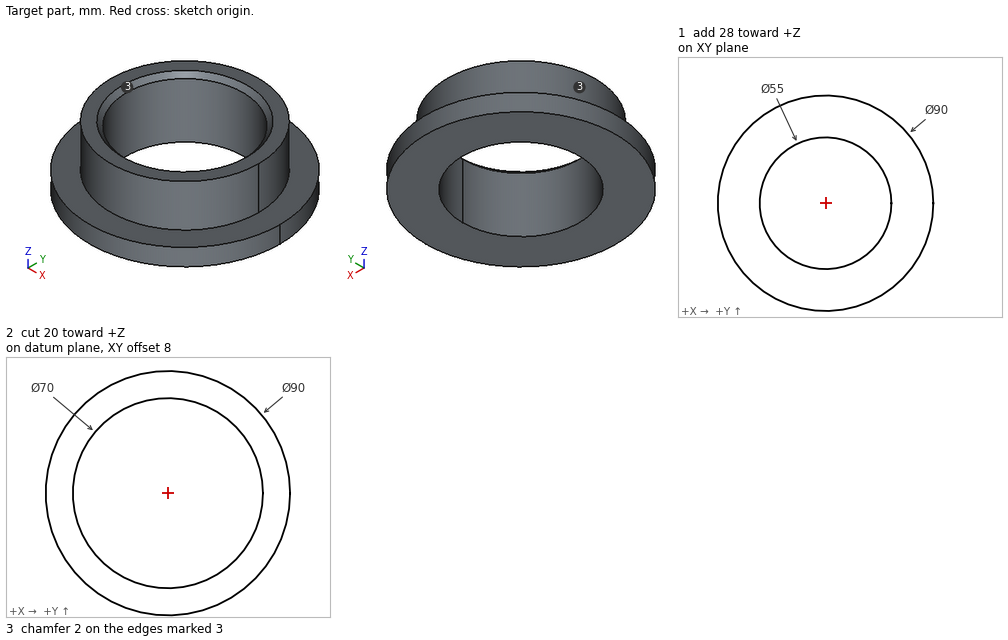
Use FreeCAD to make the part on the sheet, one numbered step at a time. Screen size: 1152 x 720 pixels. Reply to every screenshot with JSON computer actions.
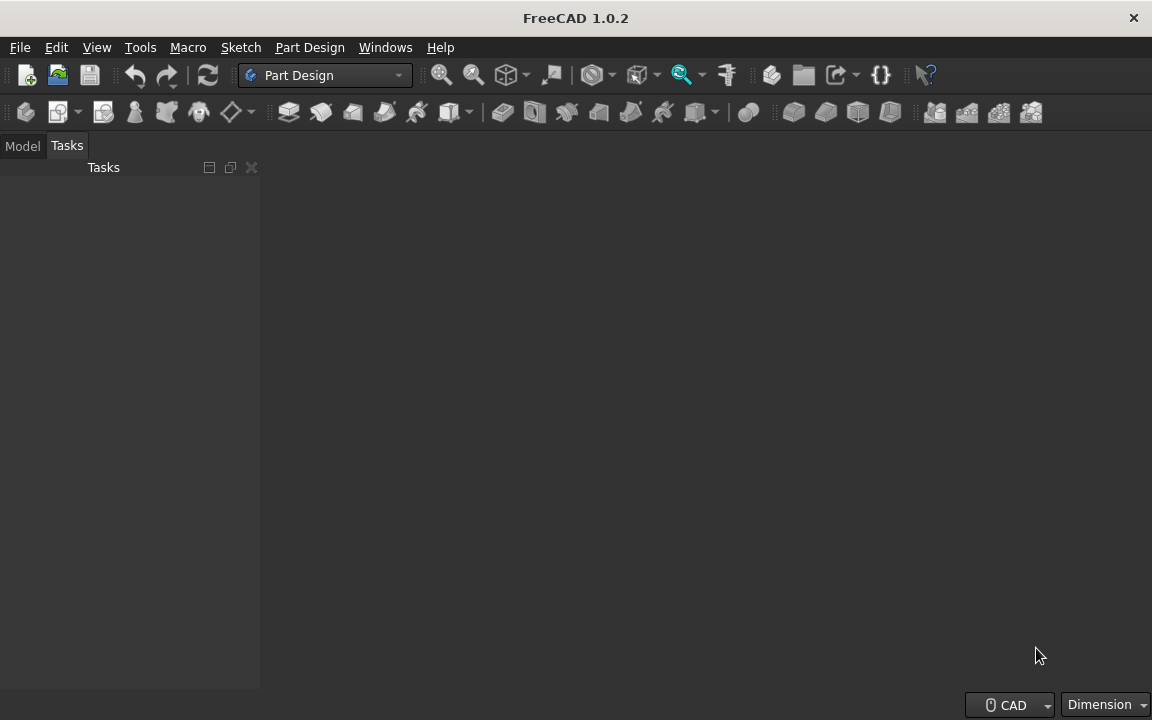
{"action": "left_click", "coordinate": [26, 76]}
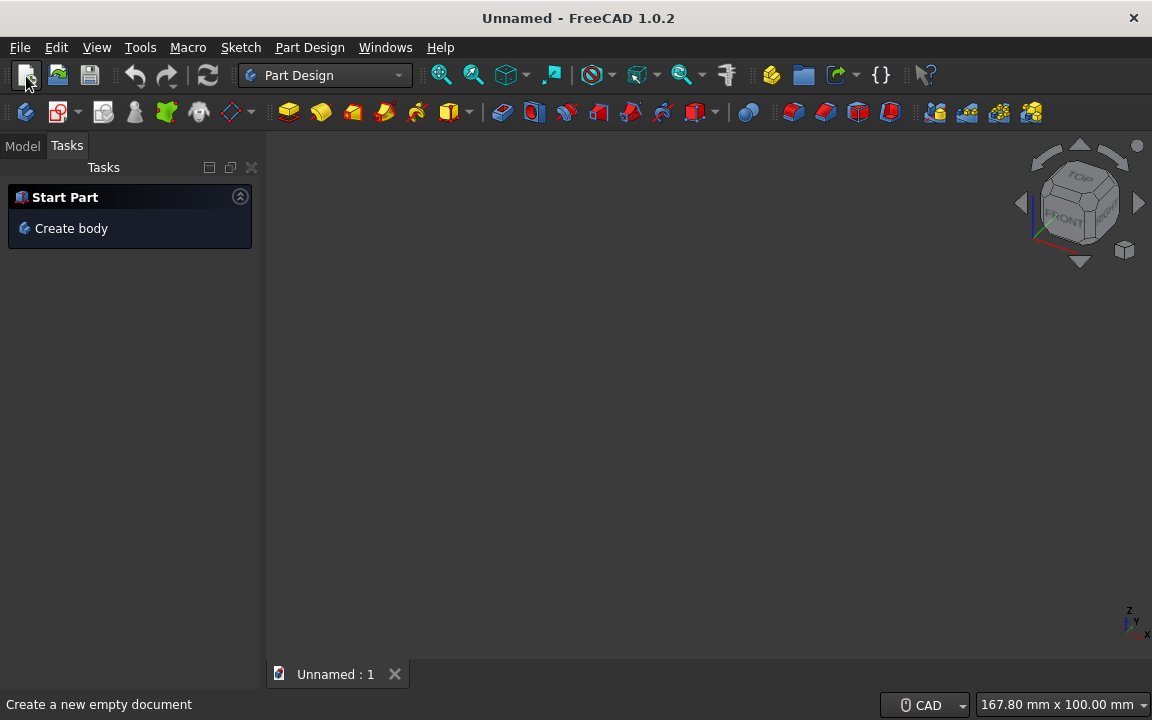
{"action": "left_click", "coordinate": [58, 112]}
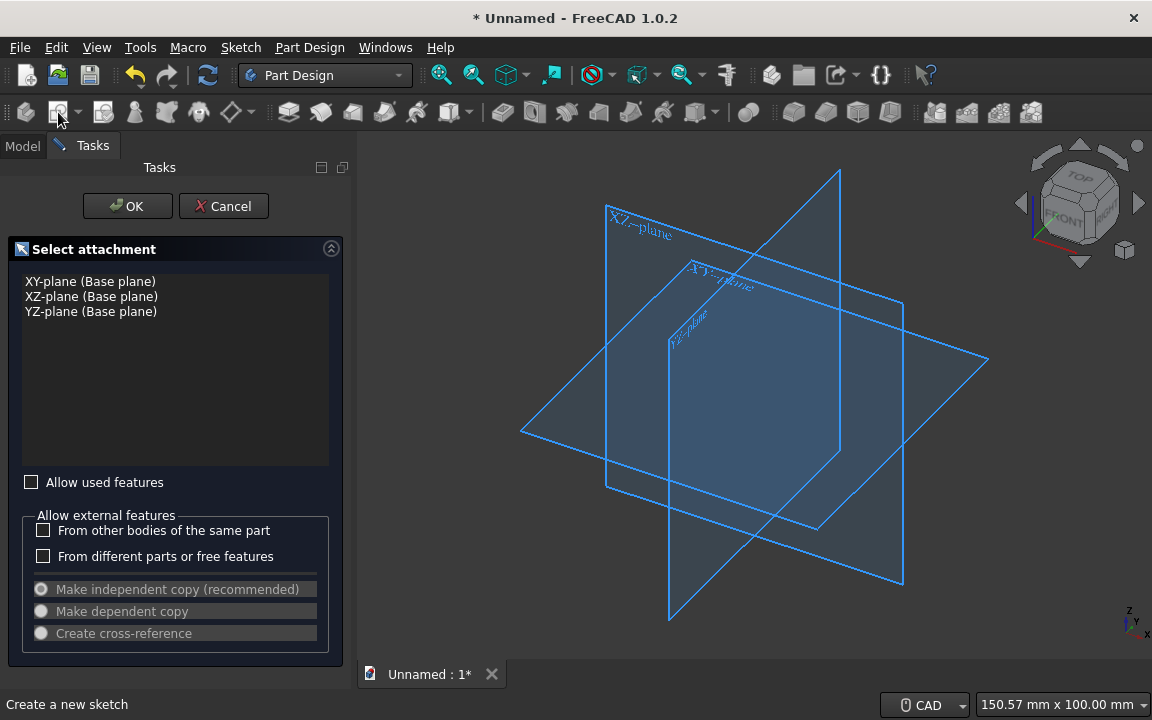
{"action": "left_click", "coordinate": [82, 282]}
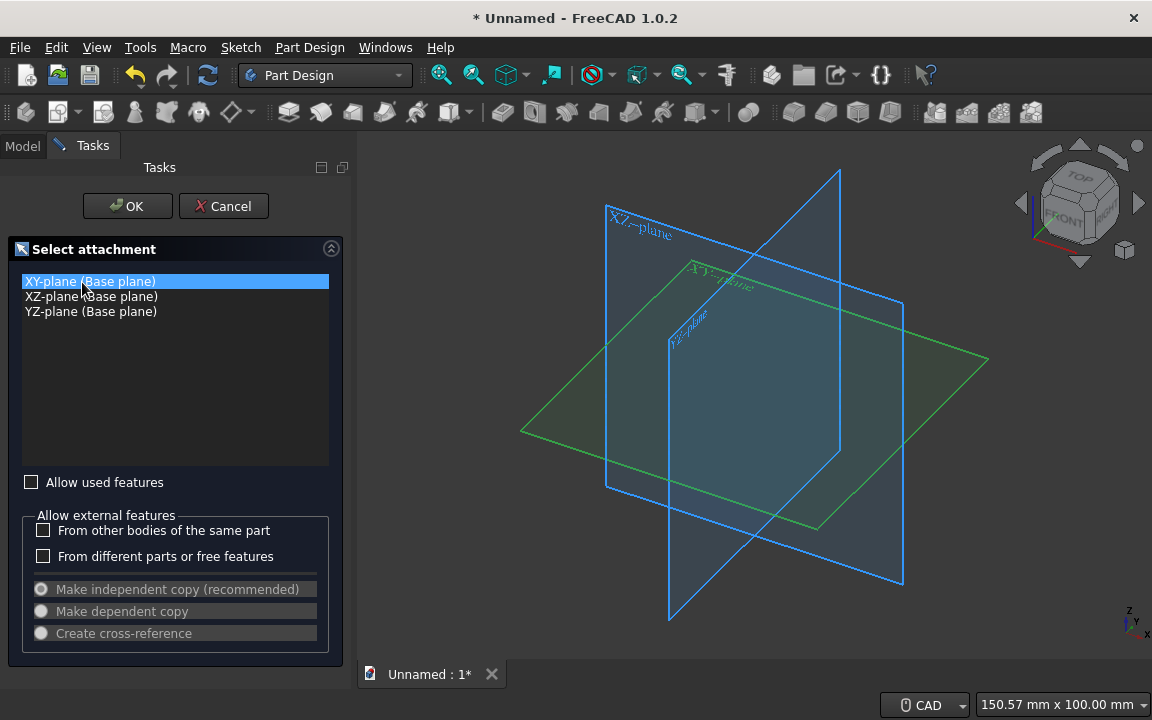
{"action": "left_click", "coordinate": [128, 206]}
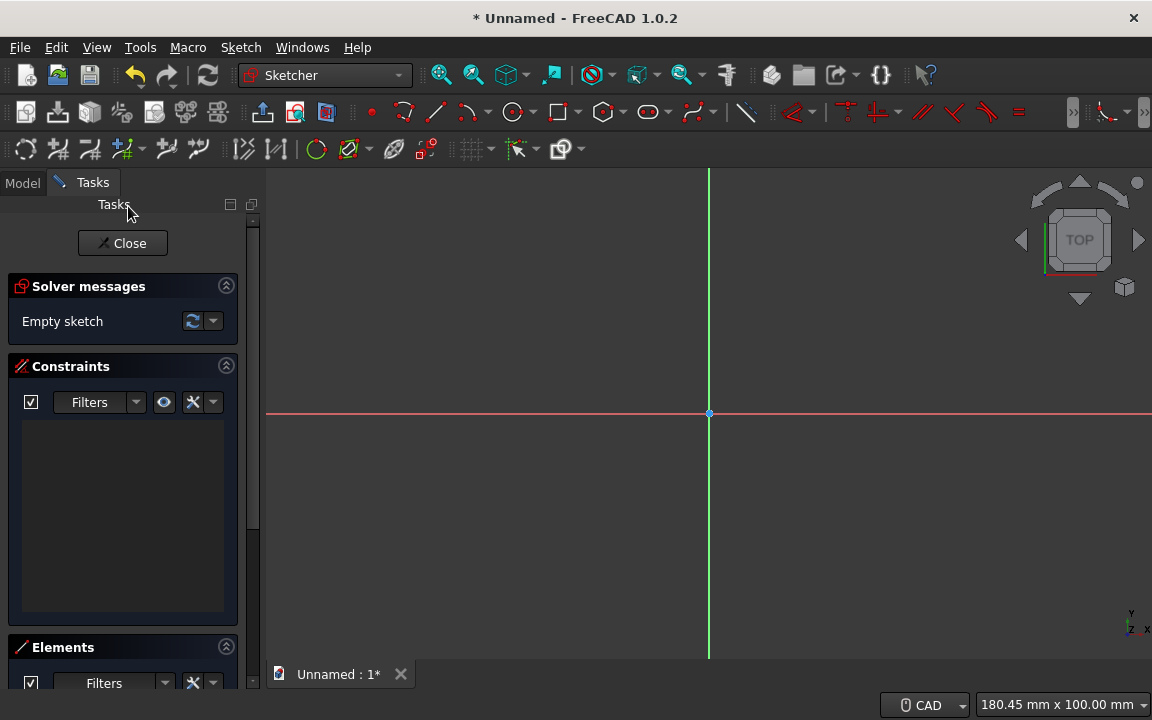
{"action": "scroll", "coordinate": [501, 414], "scroll_direction": "down", "scroll_amount": 2}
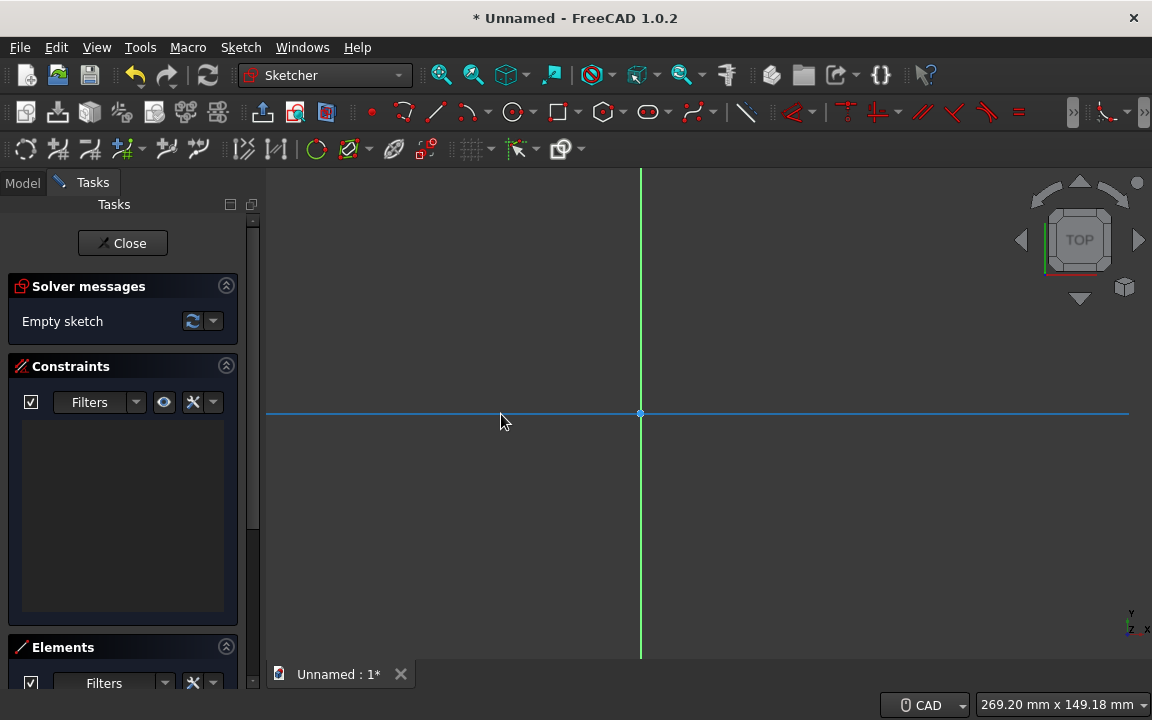
{"action": "left_click", "coordinate": [514, 112]}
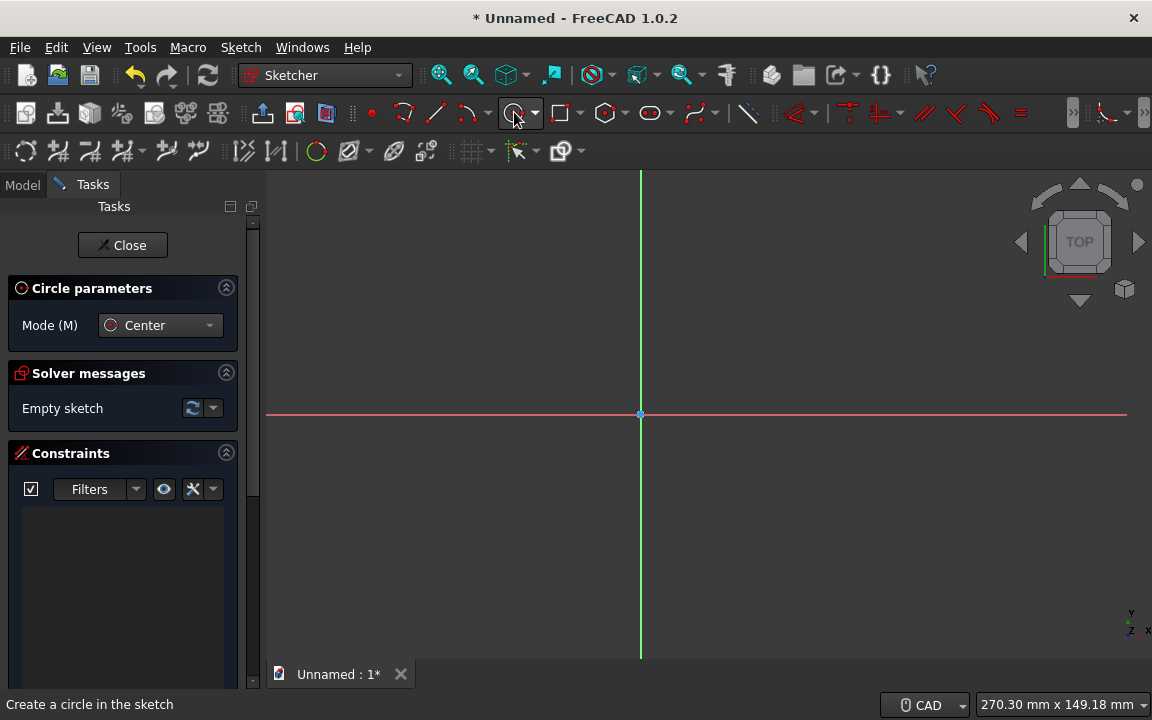
{"action": "left_click", "coordinate": [641, 415]}
{"action": "mouse_move", "coordinate": [745, 311]}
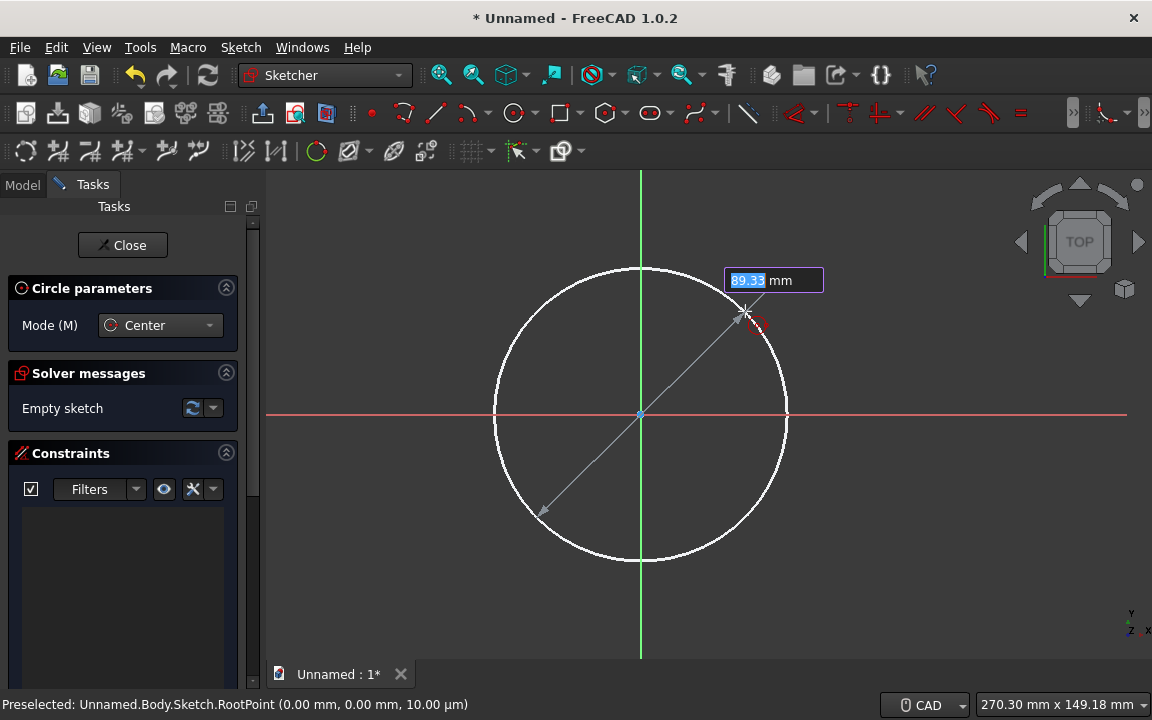
{"action": "type", "text": "90"}
{"action": "key", "text": "Return"}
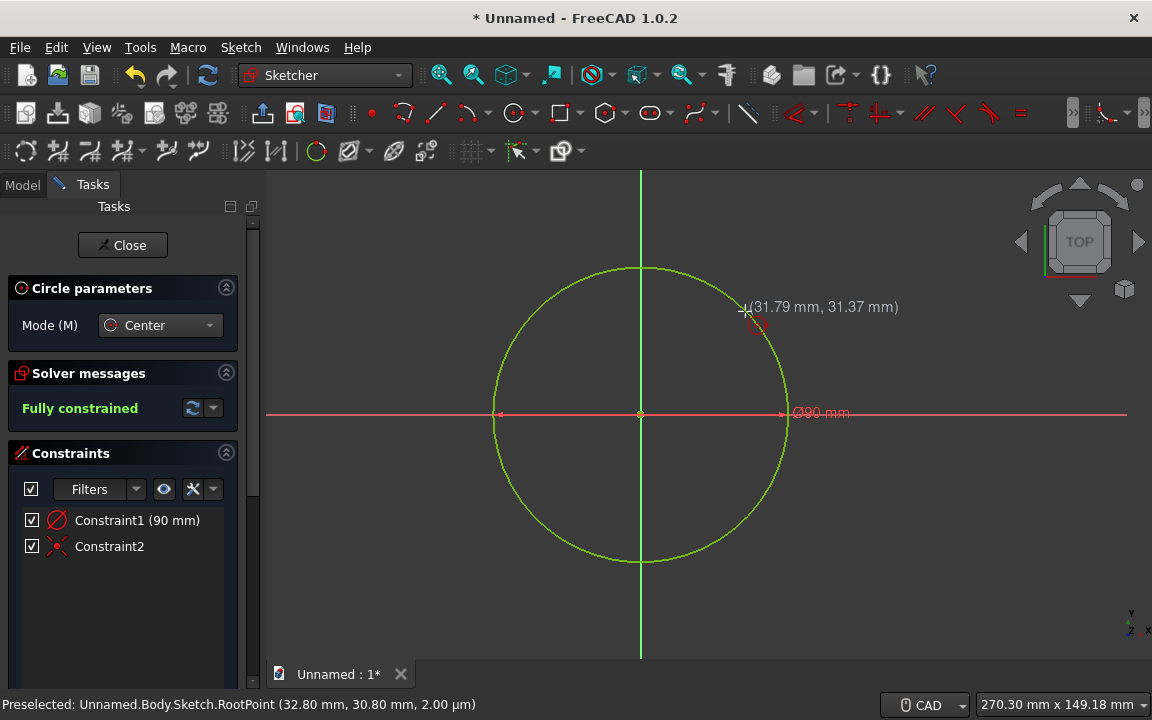
{"action": "left_click", "coordinate": [641, 415]}
{"action": "mouse_move", "coordinate": [705, 351]}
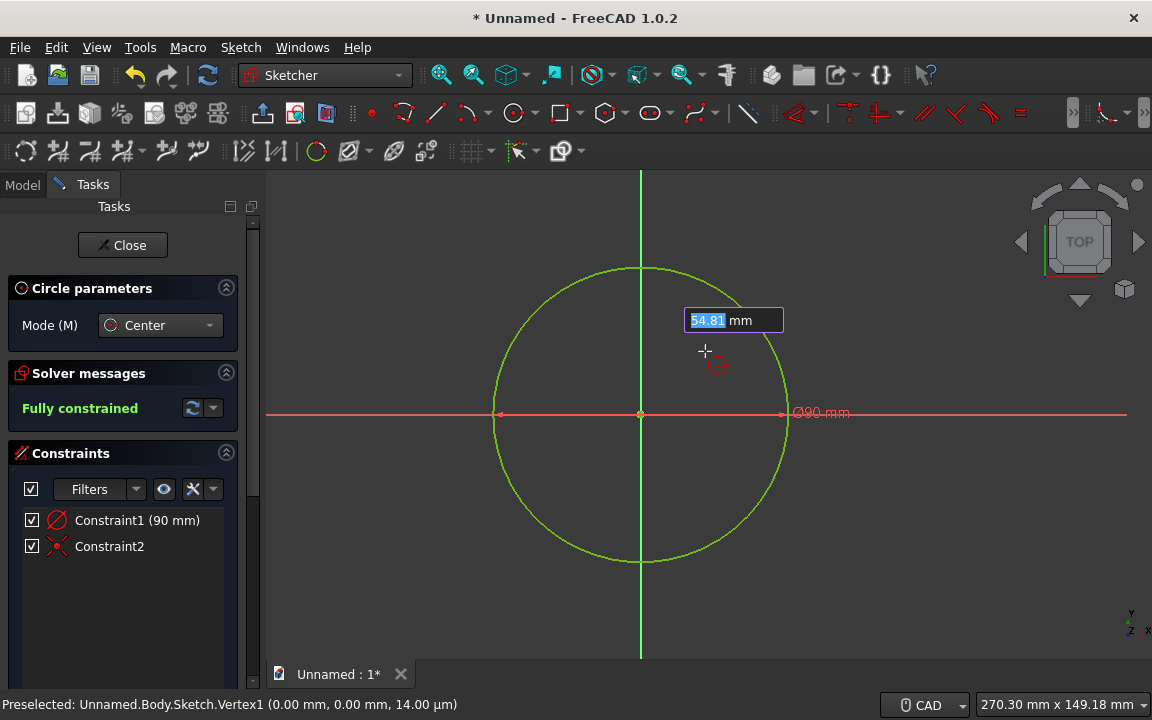
{"action": "type", "text": "55"}
{"action": "key", "text": "Return"}
{"action": "key", "text": "Escape"}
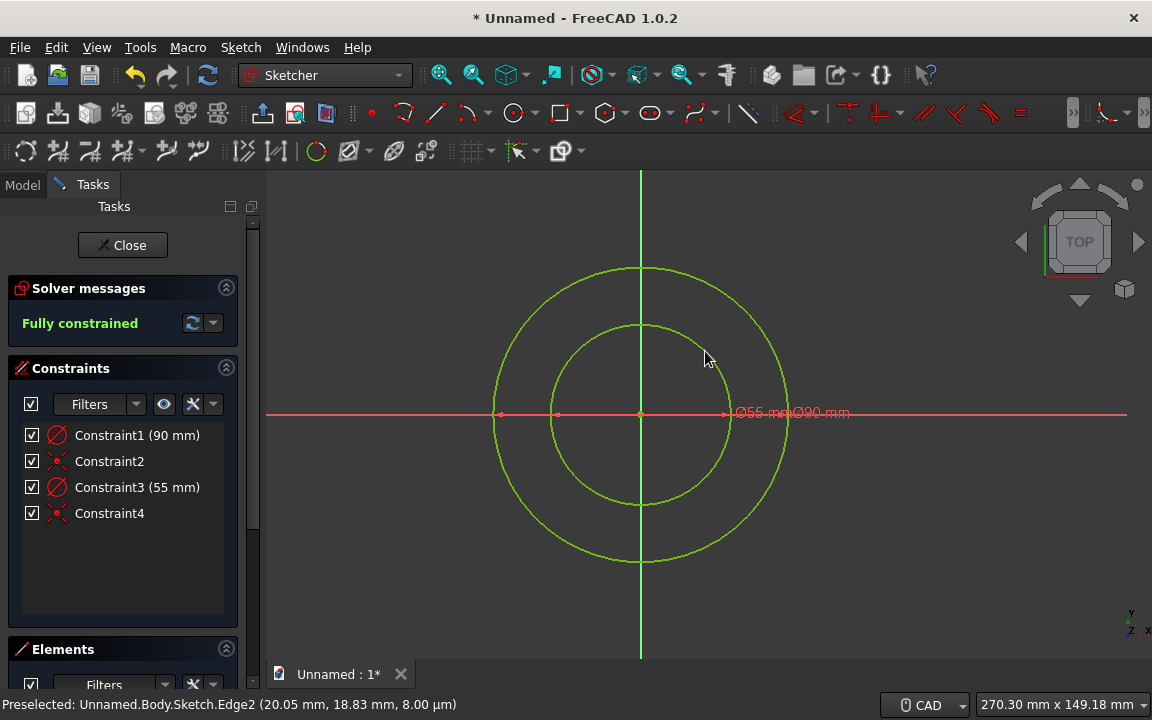
{"action": "left_click", "coordinate": [123, 245]}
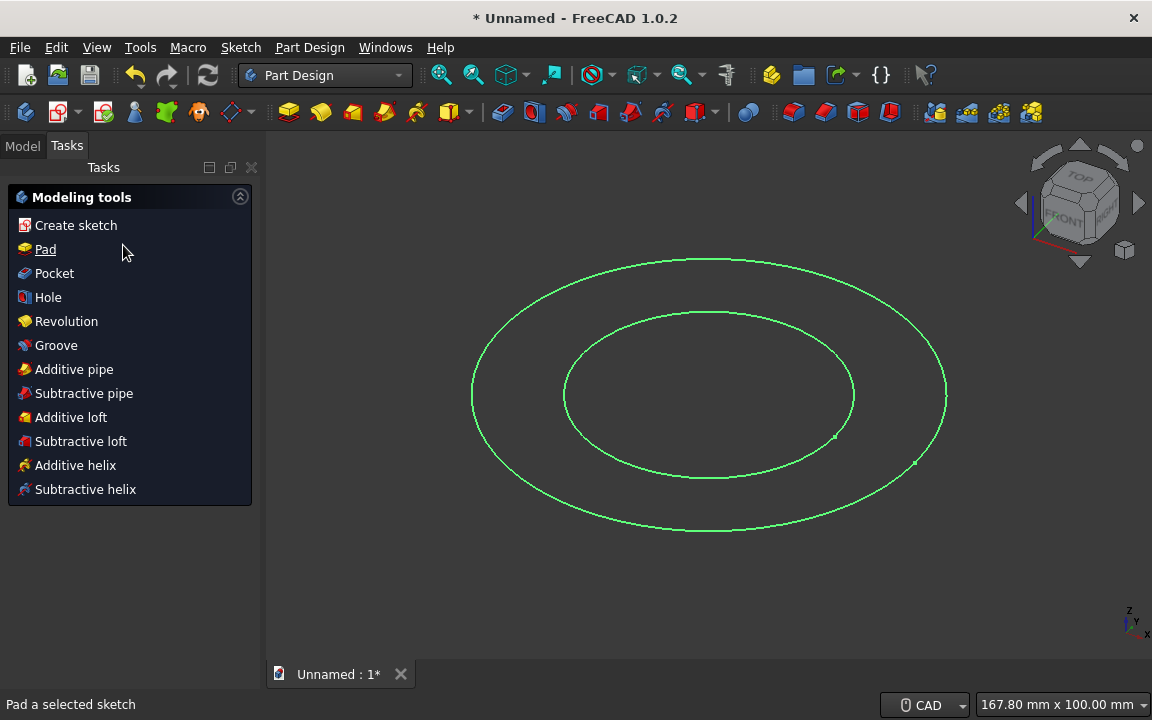
{"action": "left_click", "coordinate": [290, 112]}